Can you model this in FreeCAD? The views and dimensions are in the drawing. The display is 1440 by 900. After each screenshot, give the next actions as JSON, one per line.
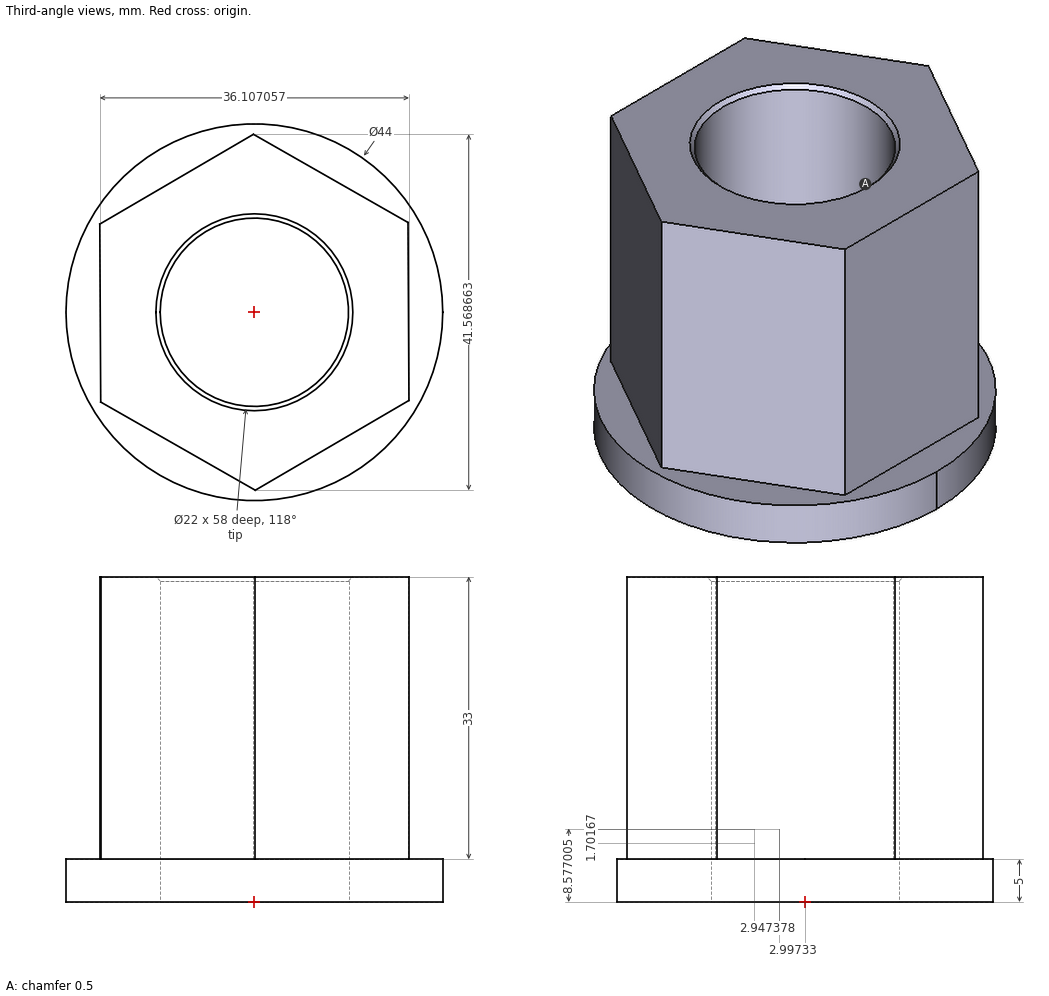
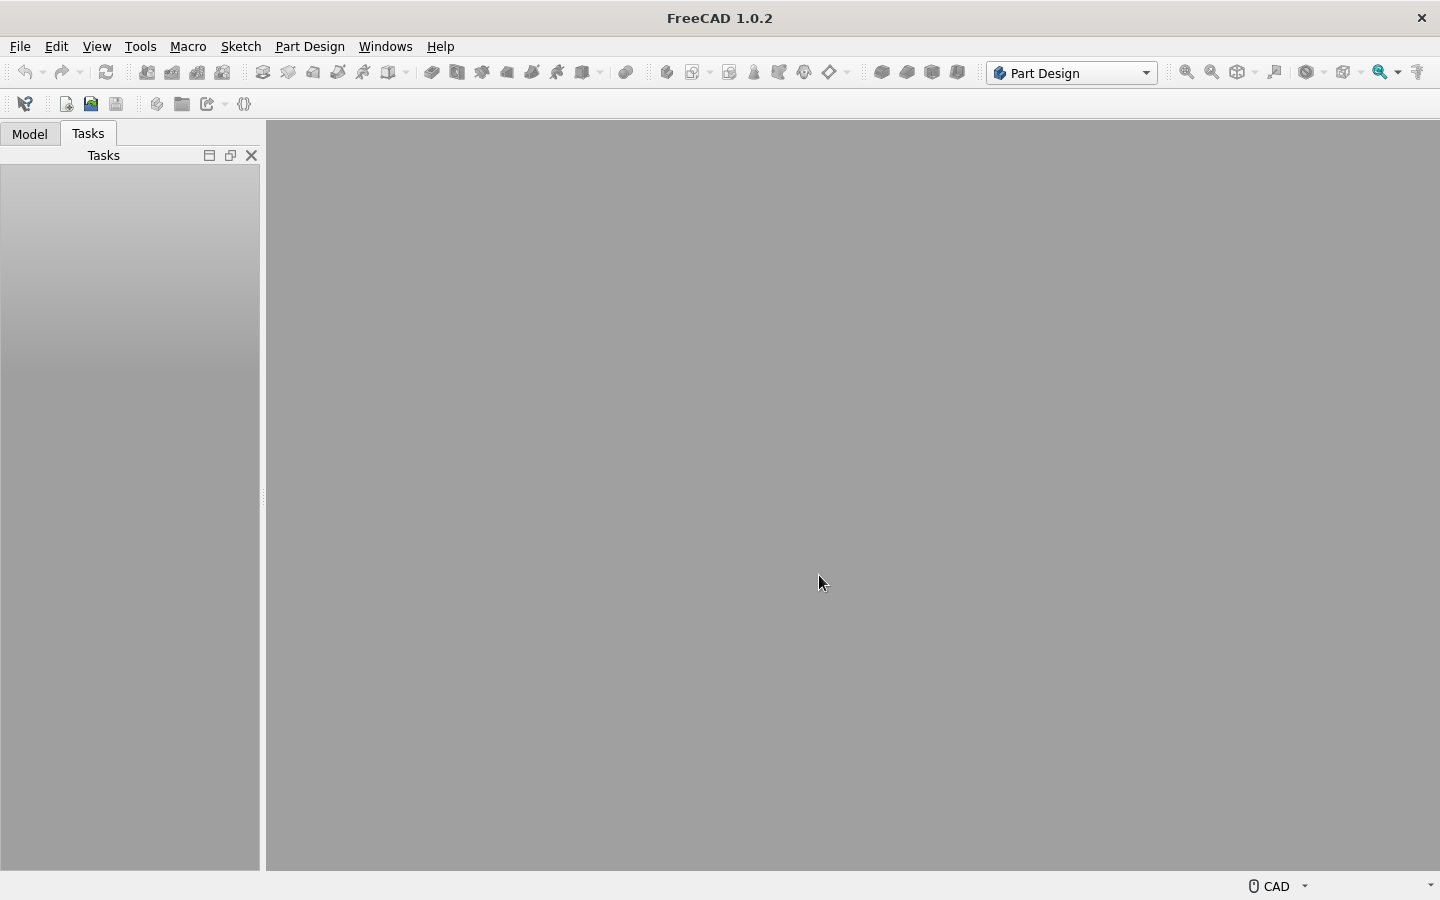
{"action": "left_click", "coordinate": [66, 104]}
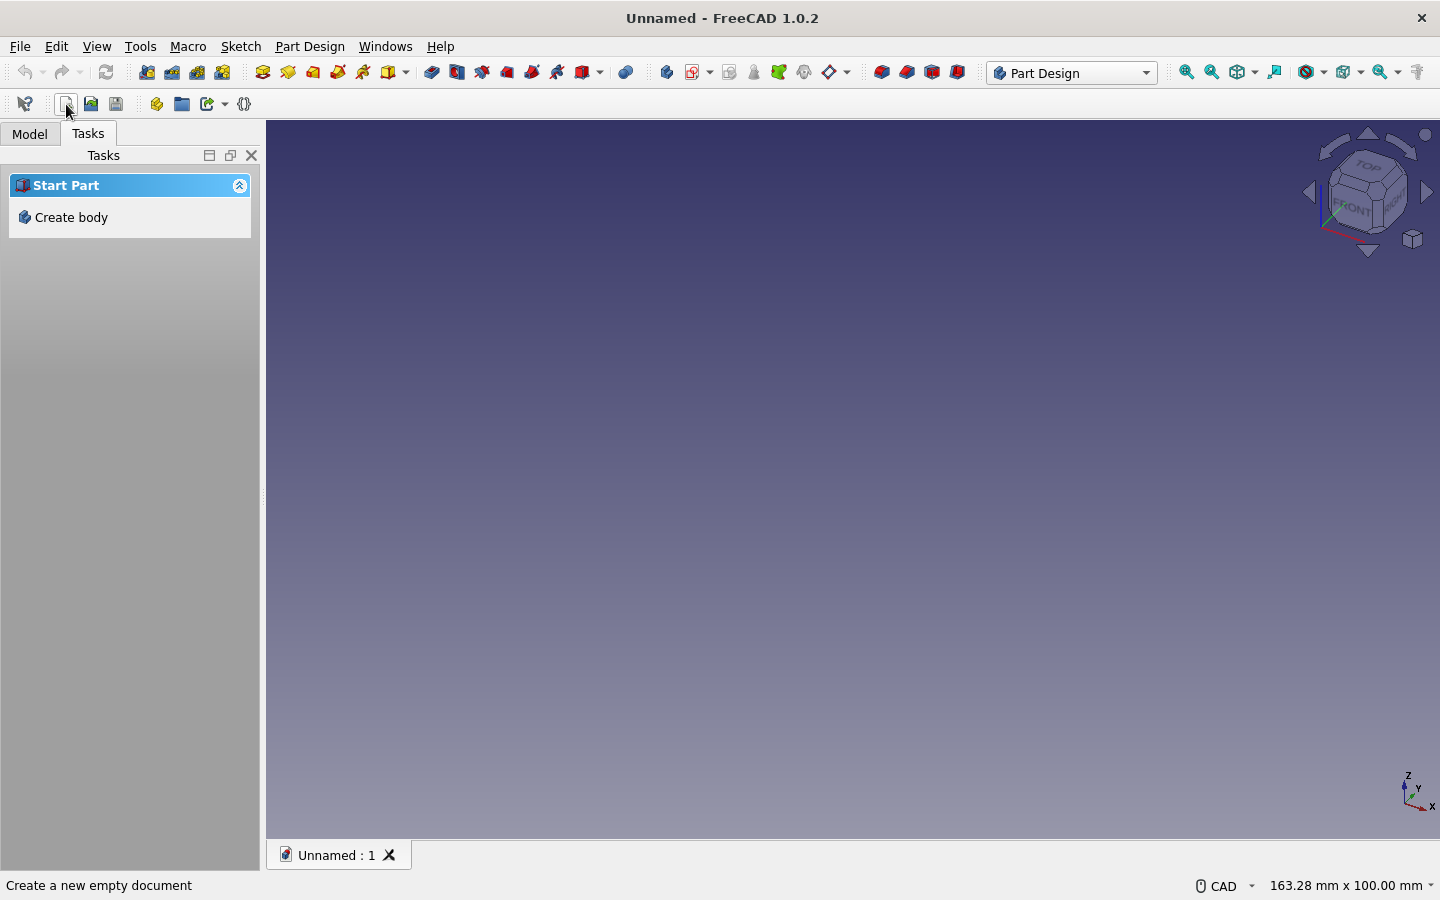
{"action": "left_click", "coordinate": [692, 72]}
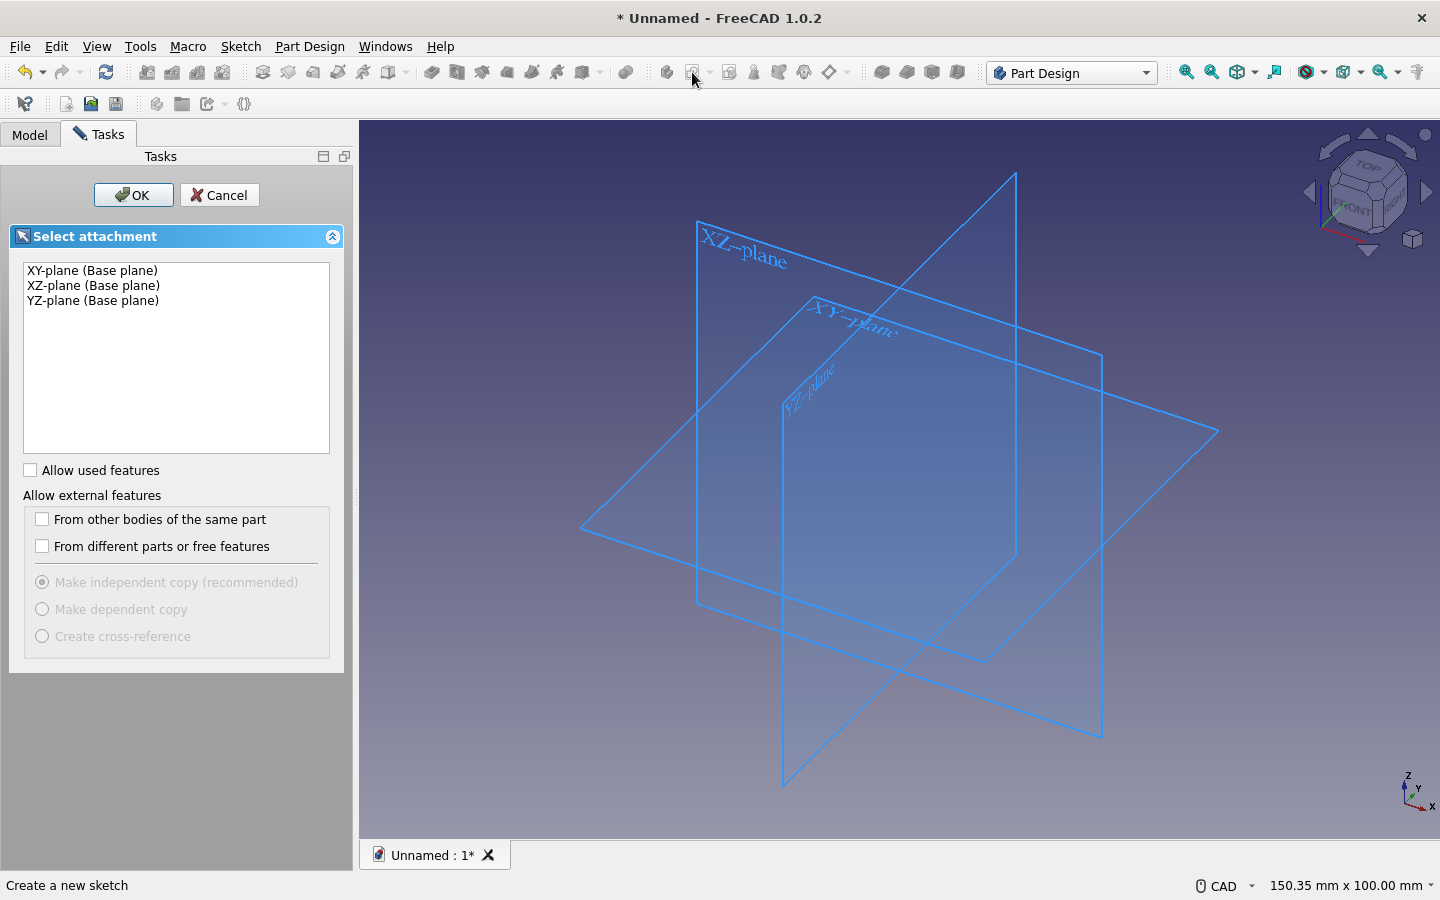
{"action": "left_click", "coordinate": [84, 270]}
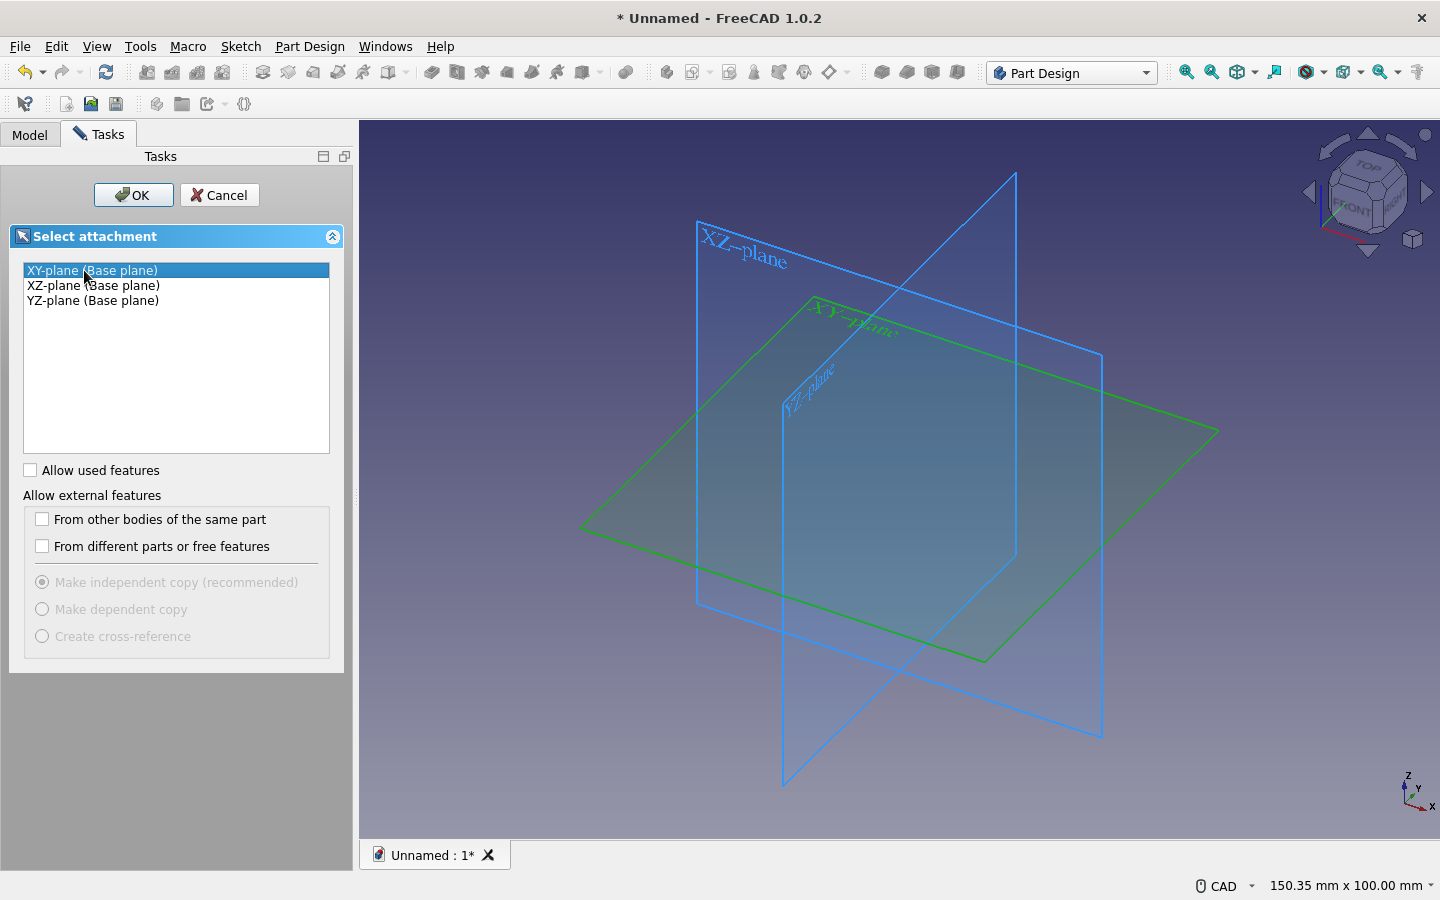
{"action": "left_click", "coordinate": [134, 195]}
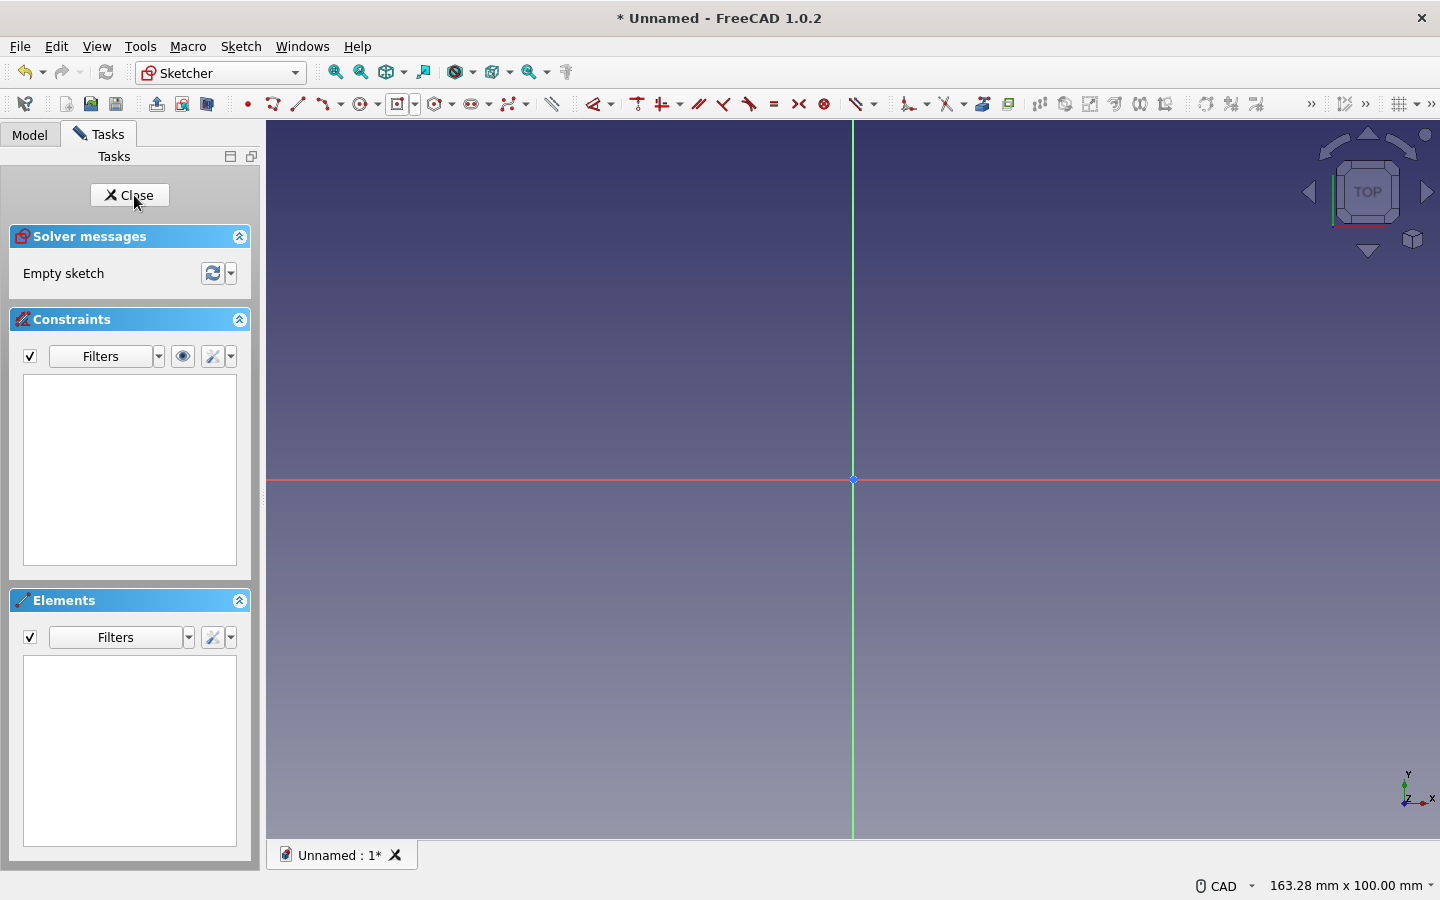
{"action": "scroll", "coordinate": [992, 480], "scroll_direction": "up", "scroll_amount": 2}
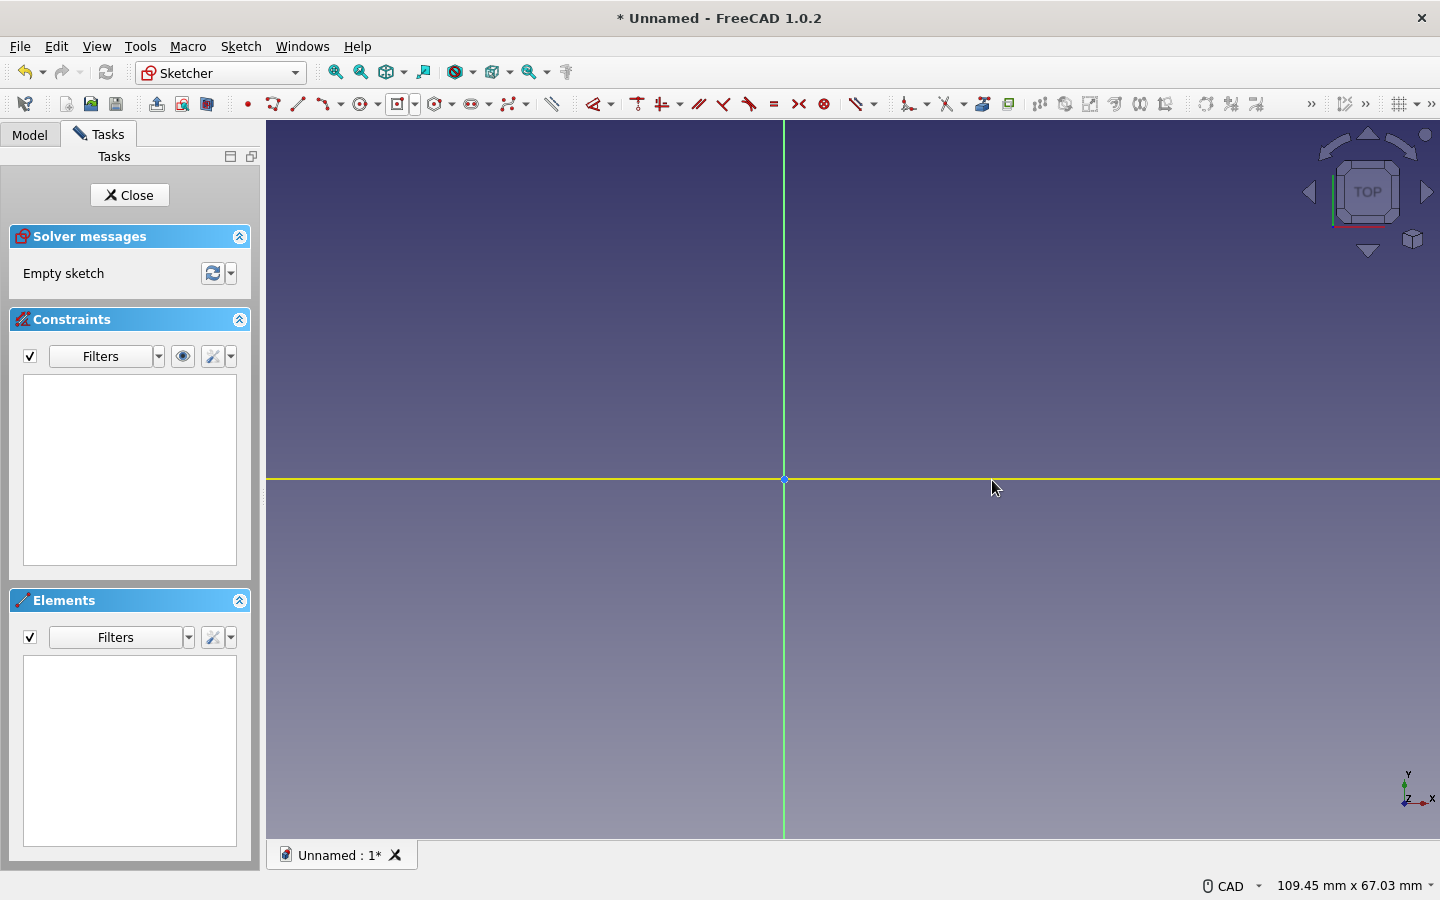
{"action": "key", "text": "g c"}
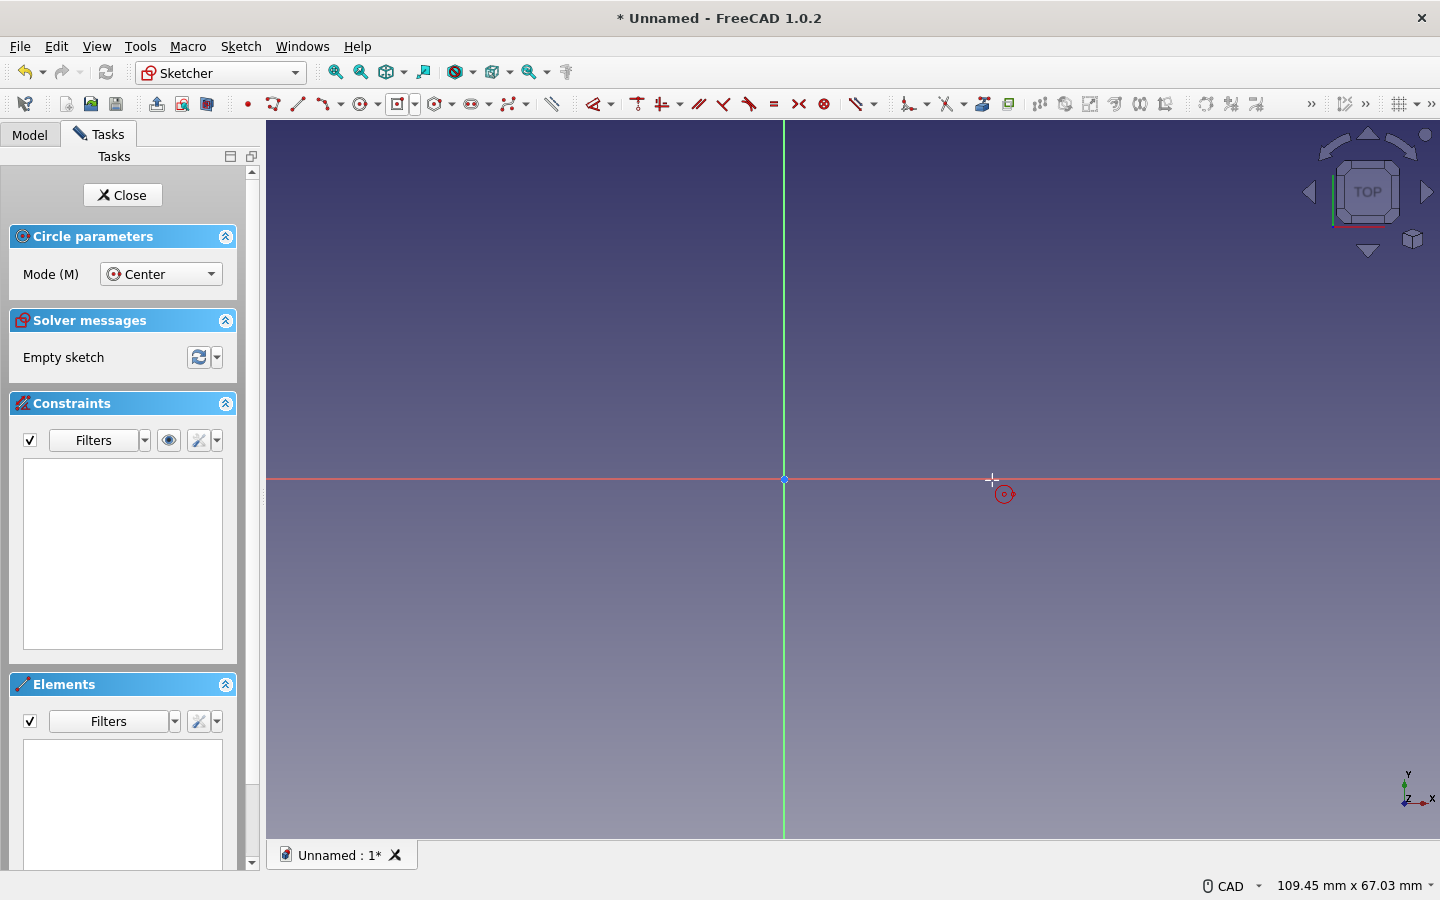
{"action": "left_click", "coordinate": [784, 479]}
{"action": "mouse_move", "coordinate": [951, 312]}